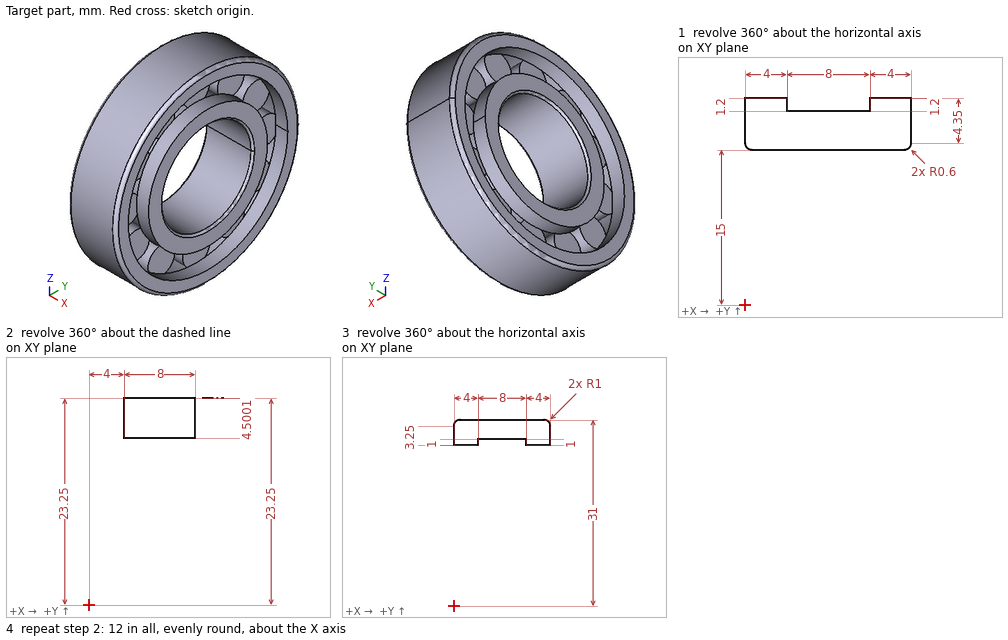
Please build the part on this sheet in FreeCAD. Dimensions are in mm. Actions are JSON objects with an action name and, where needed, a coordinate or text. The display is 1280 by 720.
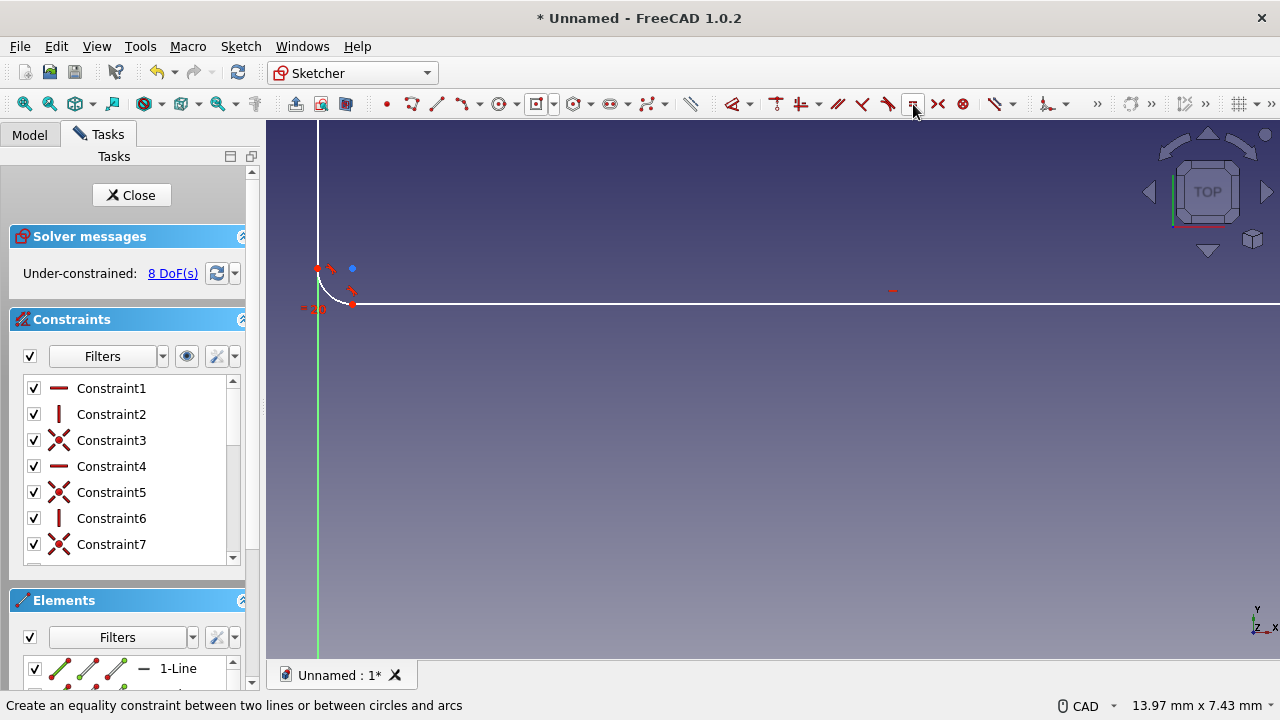
{"action": "left_click", "coordinate": [732, 104]}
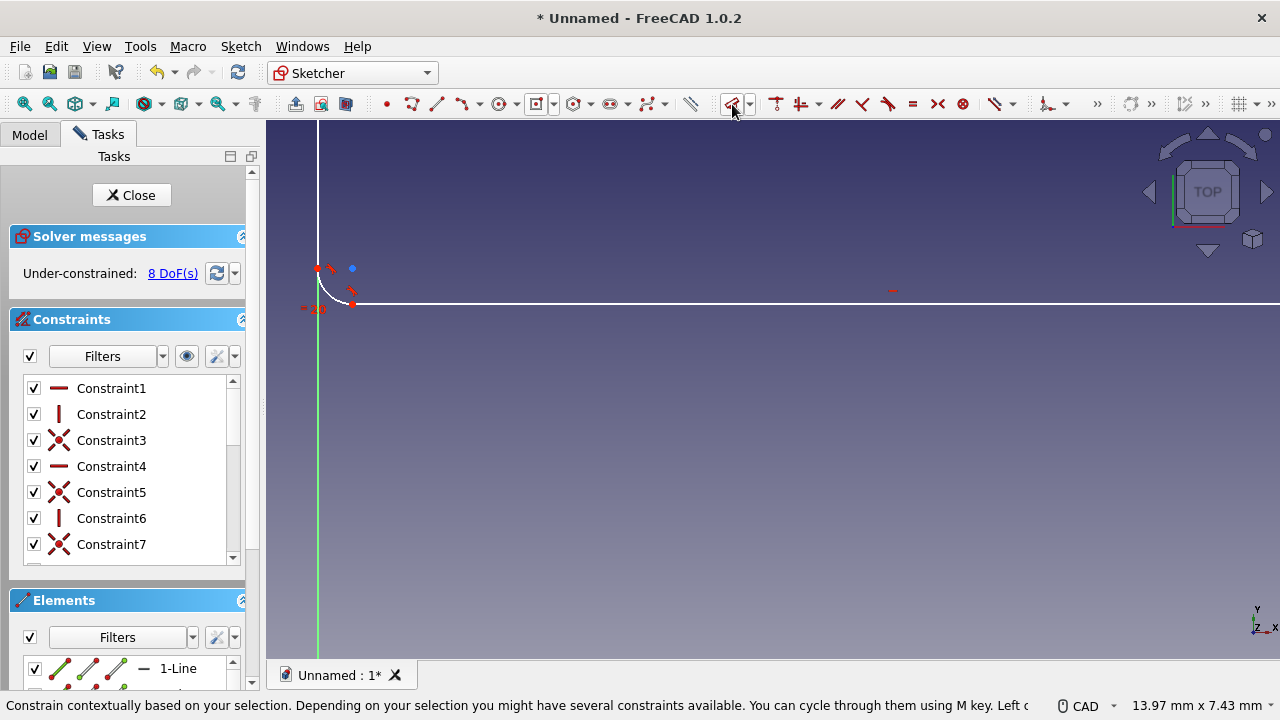
{"action": "scroll", "coordinate": [641, 299], "scroll_direction": "down", "scroll_amount": 7}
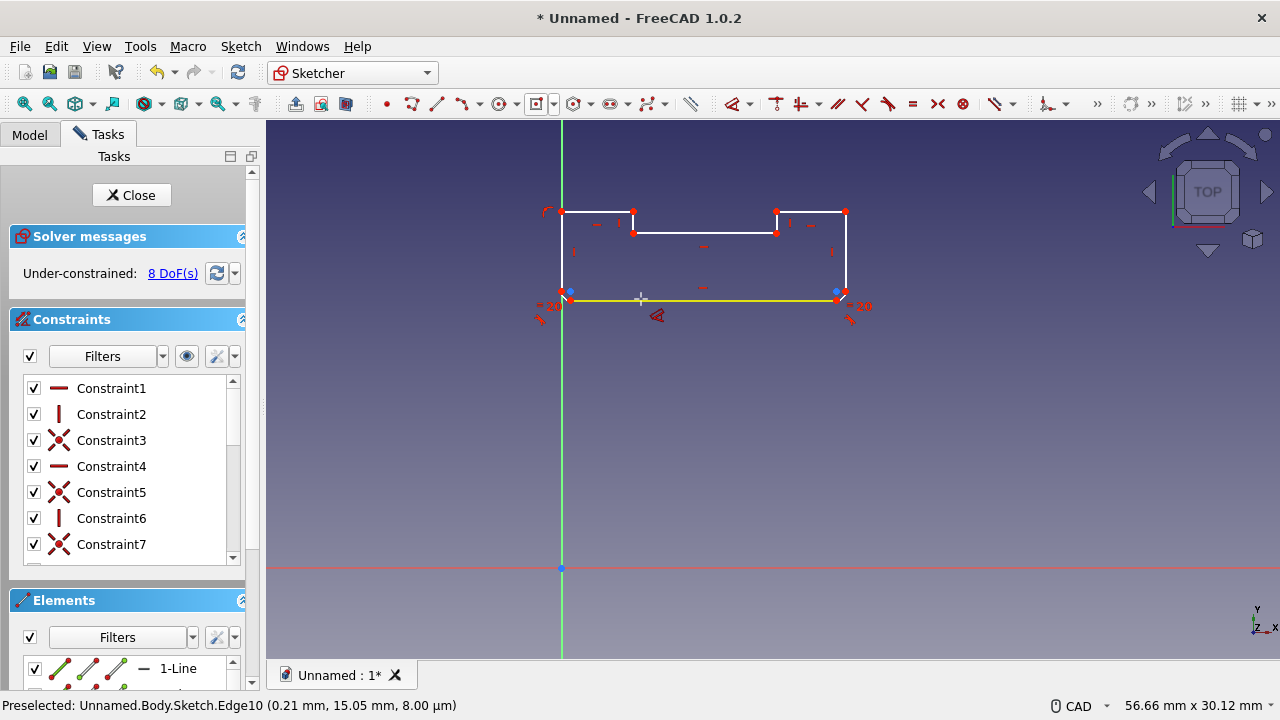
{"action": "scroll", "coordinate": [841, 300], "scroll_direction": "up", "scroll_amount": 7}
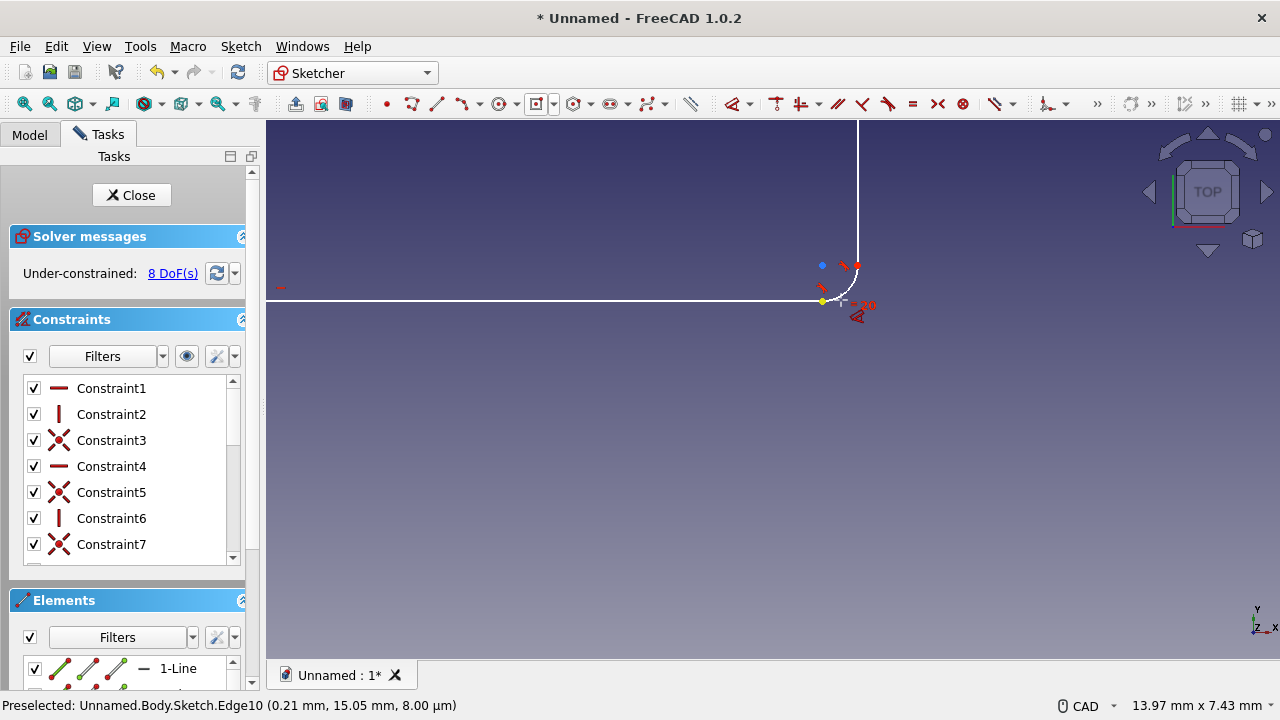
{"action": "left_click", "coordinate": [839, 297]}
{"action": "left_click", "coordinate": [854, 325]}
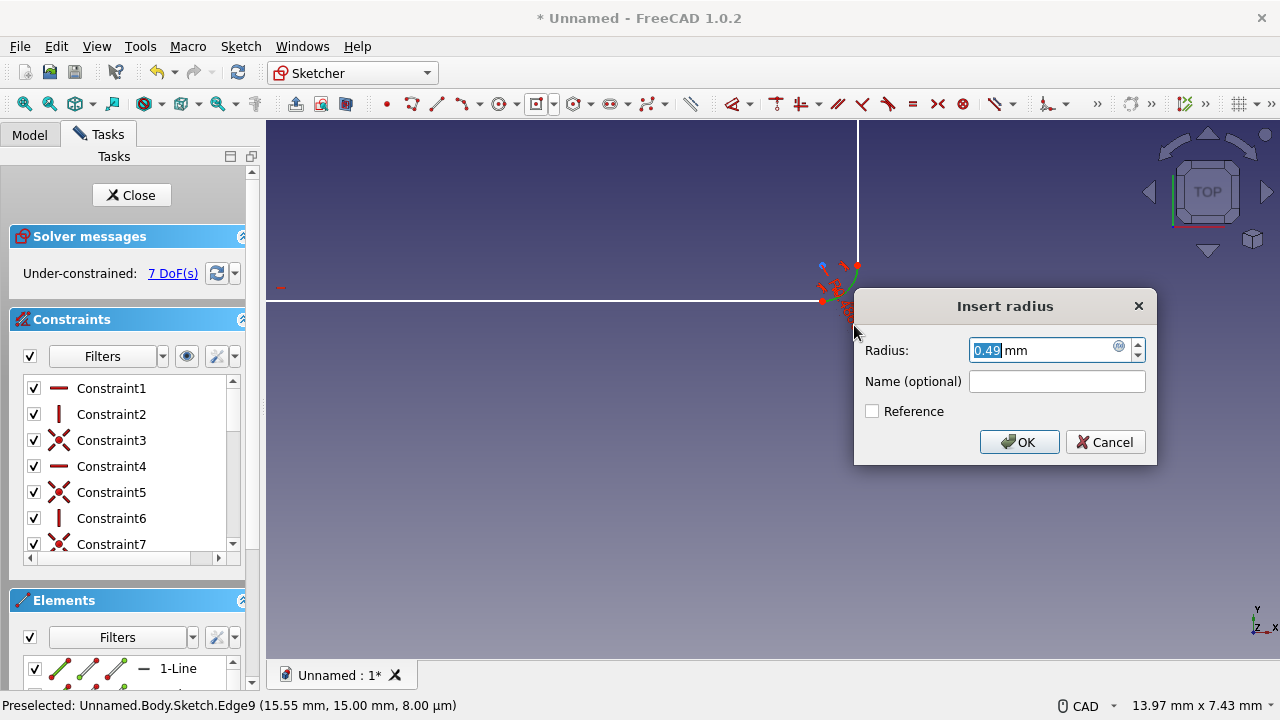
{"action": "type", "text": "0.6"}
{"action": "key", "text": "Return"}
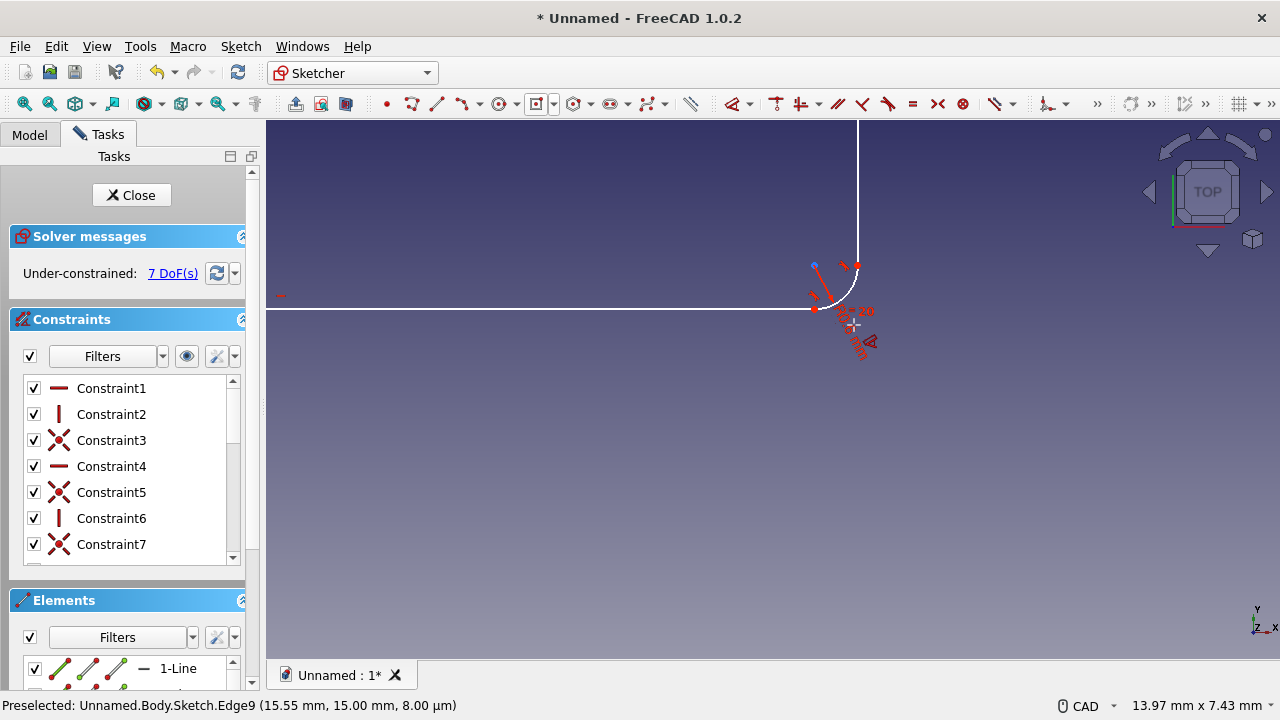
{"action": "scroll", "coordinate": [841, 300], "scroll_direction": "down", "scroll_amount": 7}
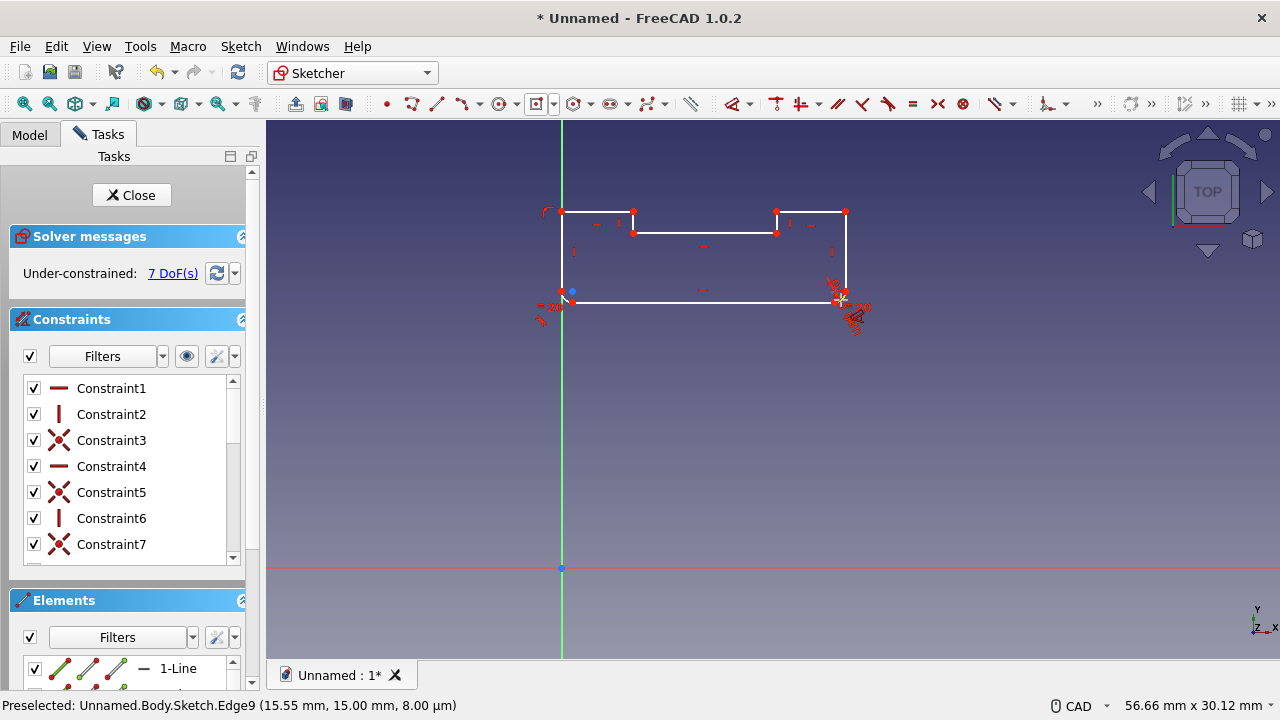
{"action": "left_click", "coordinate": [825, 212]}
{"action": "left_click", "coordinate": [811, 178]}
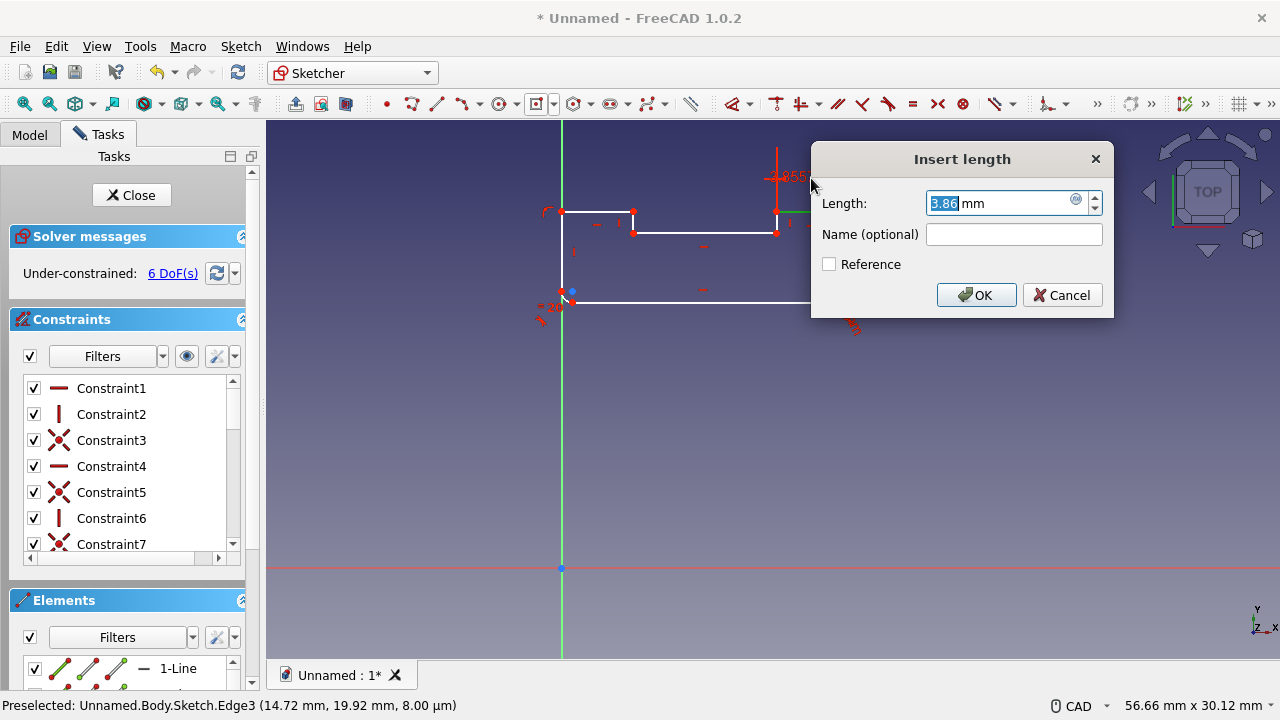
{"action": "type", "text": "4"}
{"action": "key", "text": "Return"}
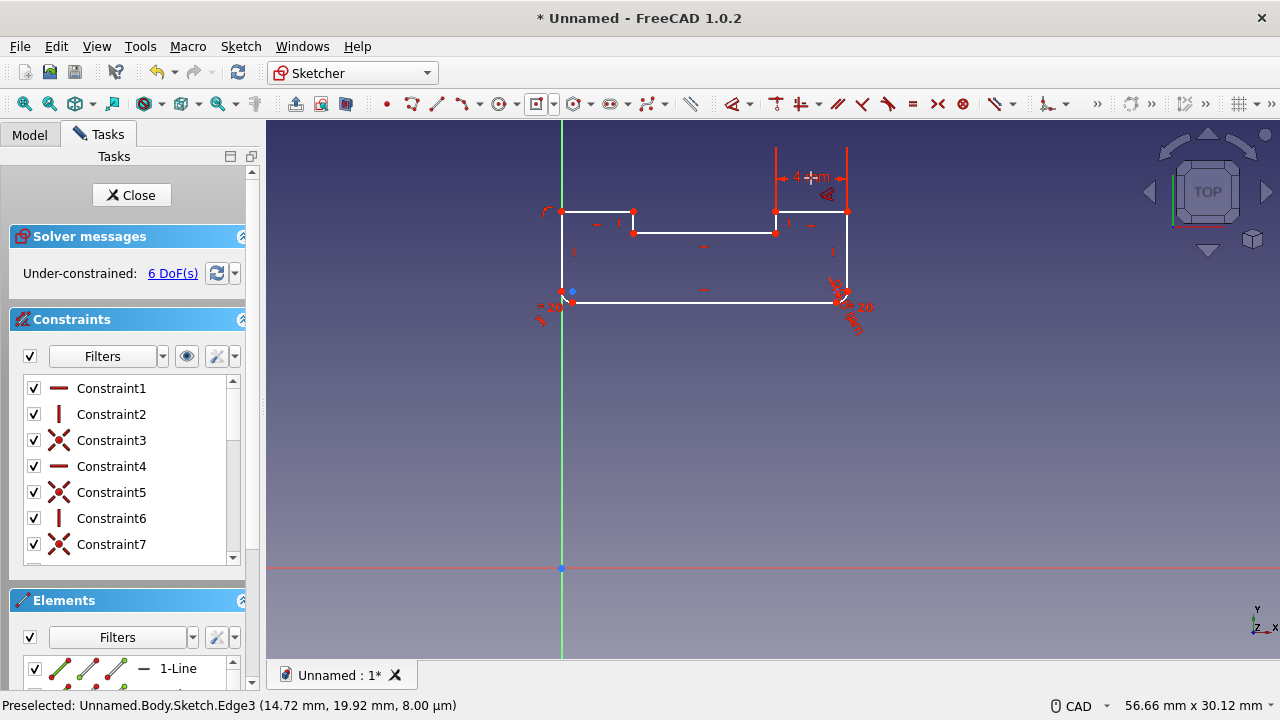
{"action": "left_click", "coordinate": [733, 233]}
{"action": "left_click", "coordinate": [704, 199]}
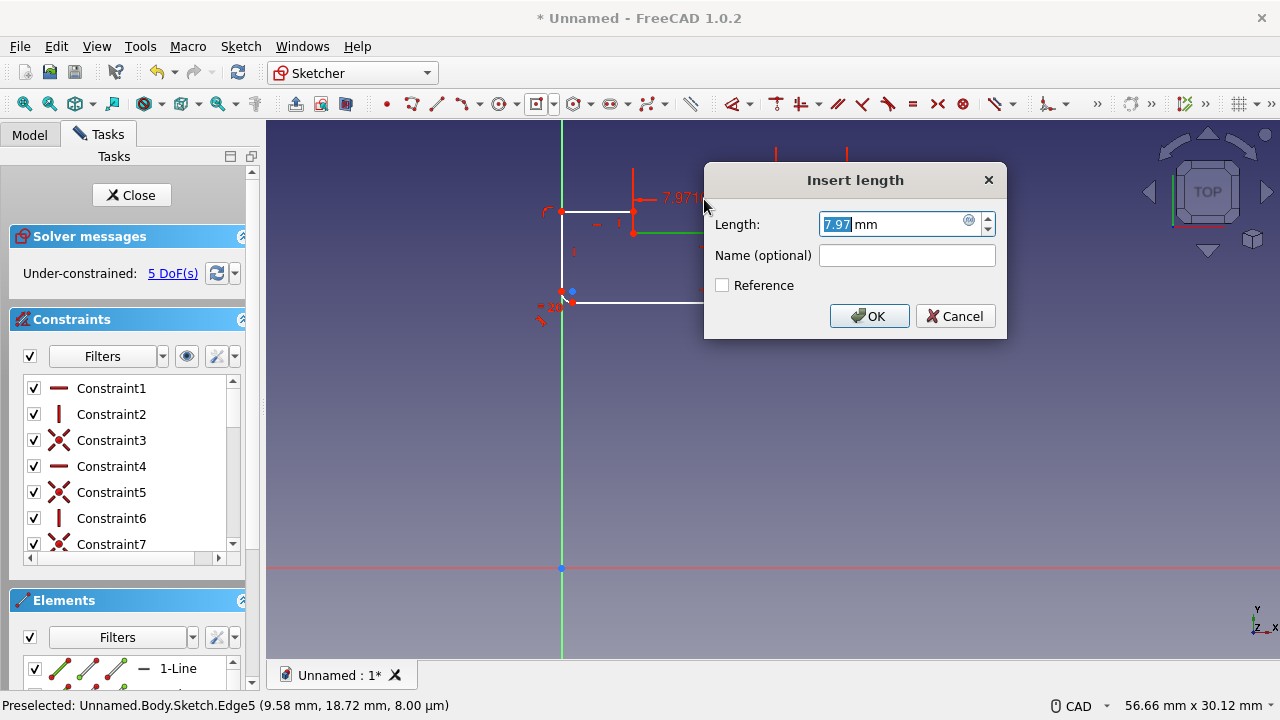
{"action": "type", "text": "8"}
{"action": "key", "text": "Return"}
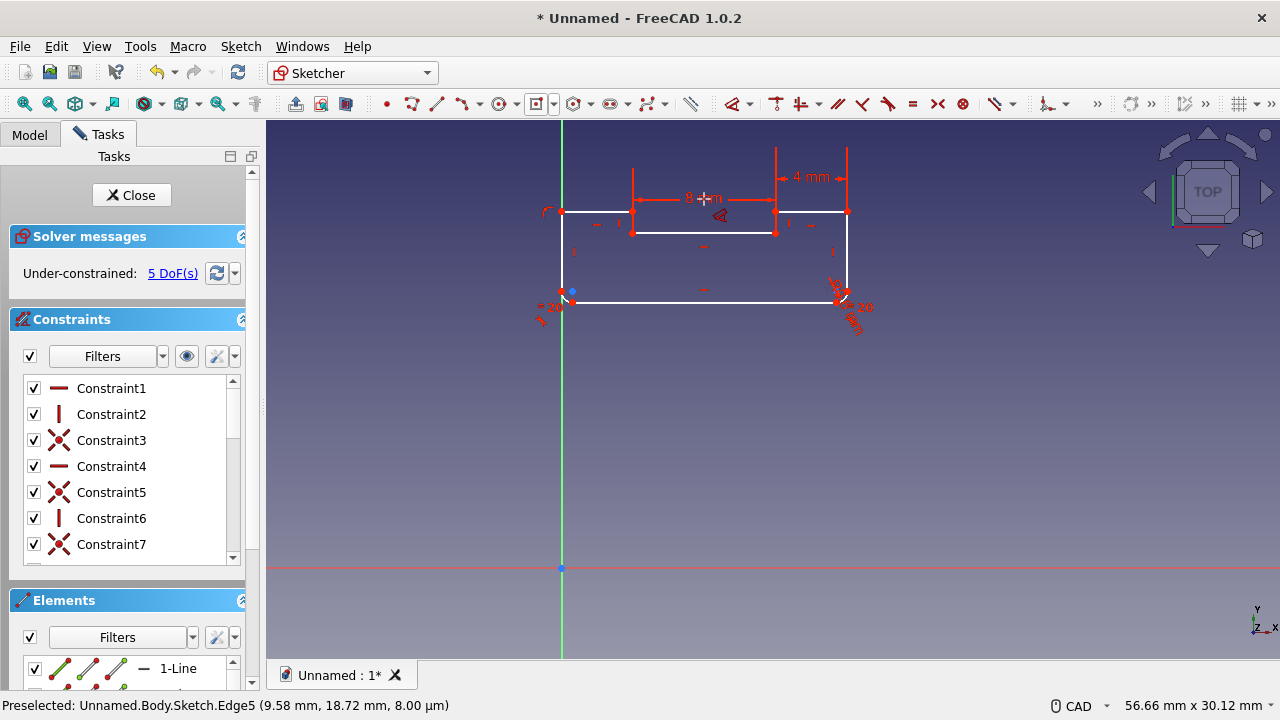
{"action": "left_click", "coordinate": [611, 212]}
{"action": "left_click", "coordinate": [597, 178]}